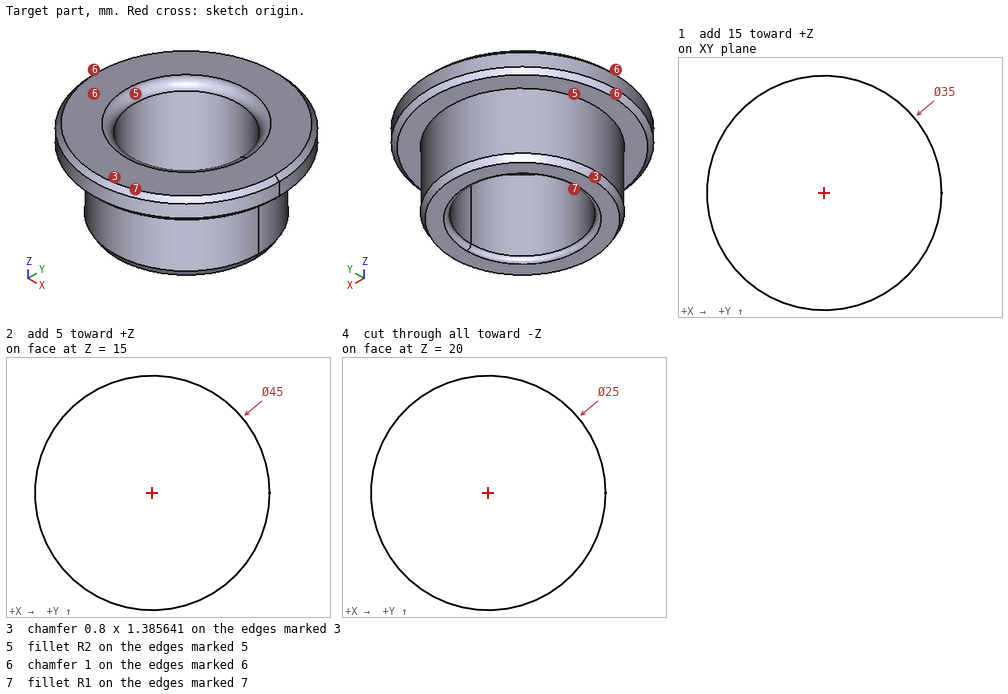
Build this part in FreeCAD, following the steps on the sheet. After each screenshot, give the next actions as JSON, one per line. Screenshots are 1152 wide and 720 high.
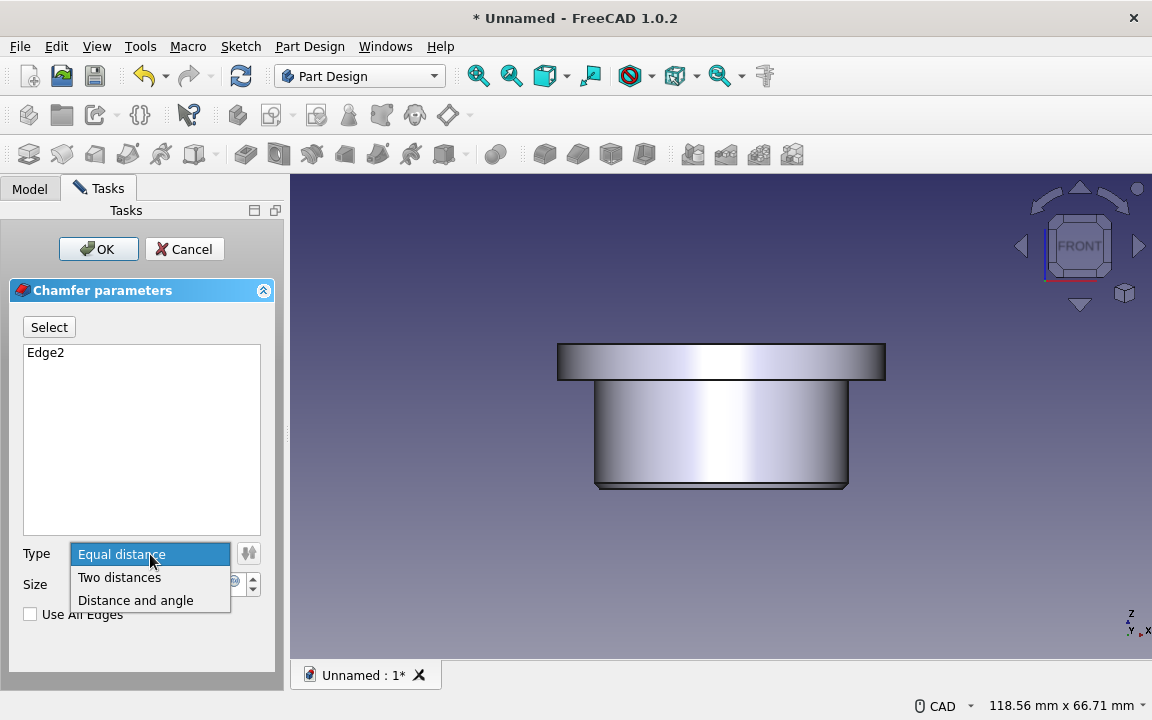
{"action": "left_click", "coordinate": [148, 578]}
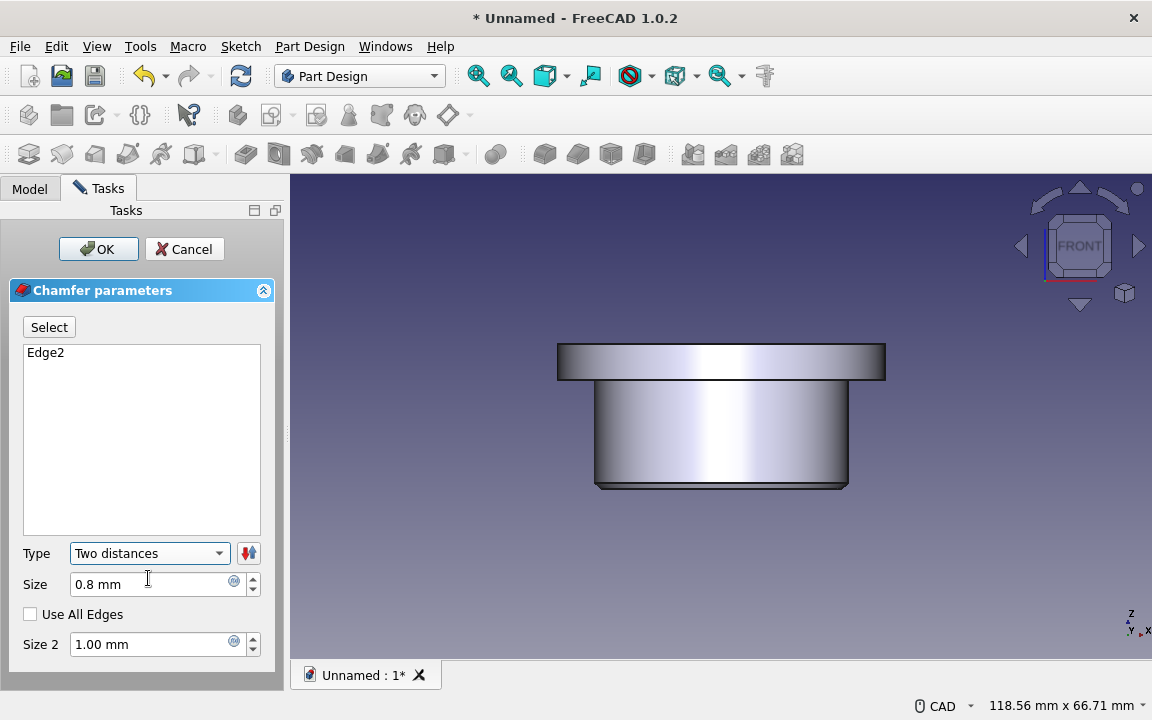
{"action": "triple_click", "coordinate": [158, 644]}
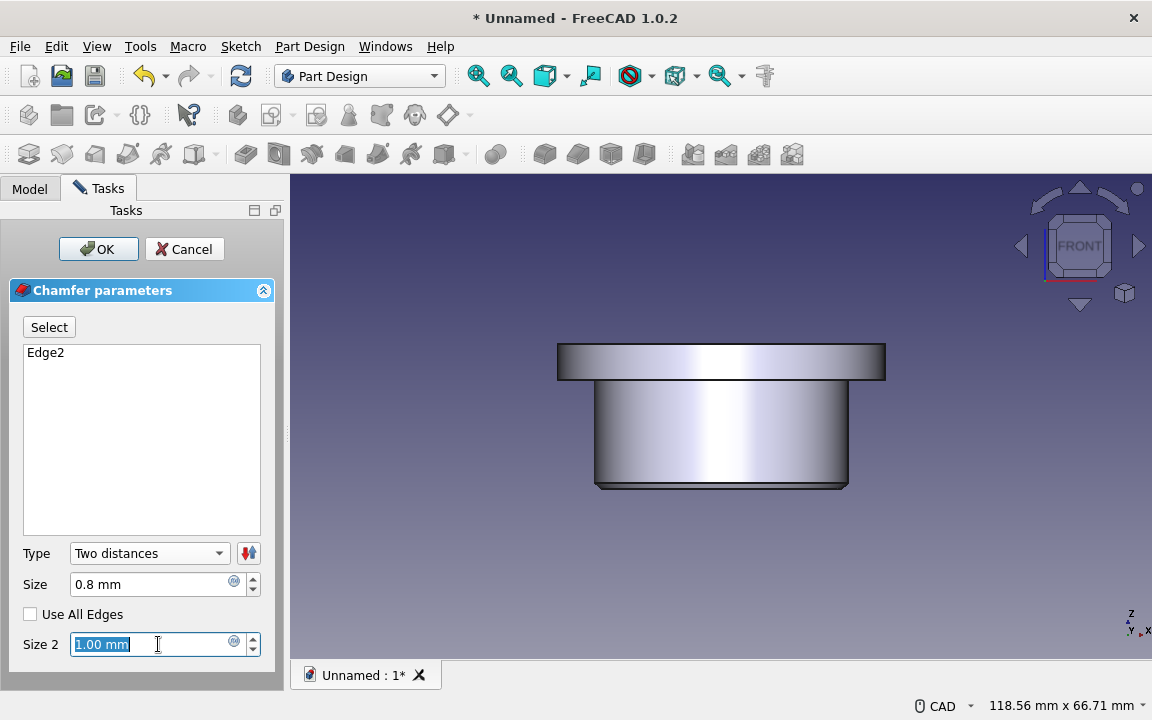
{"action": "type", "text": "1.385641"}
{"action": "key", "text": "Tab"}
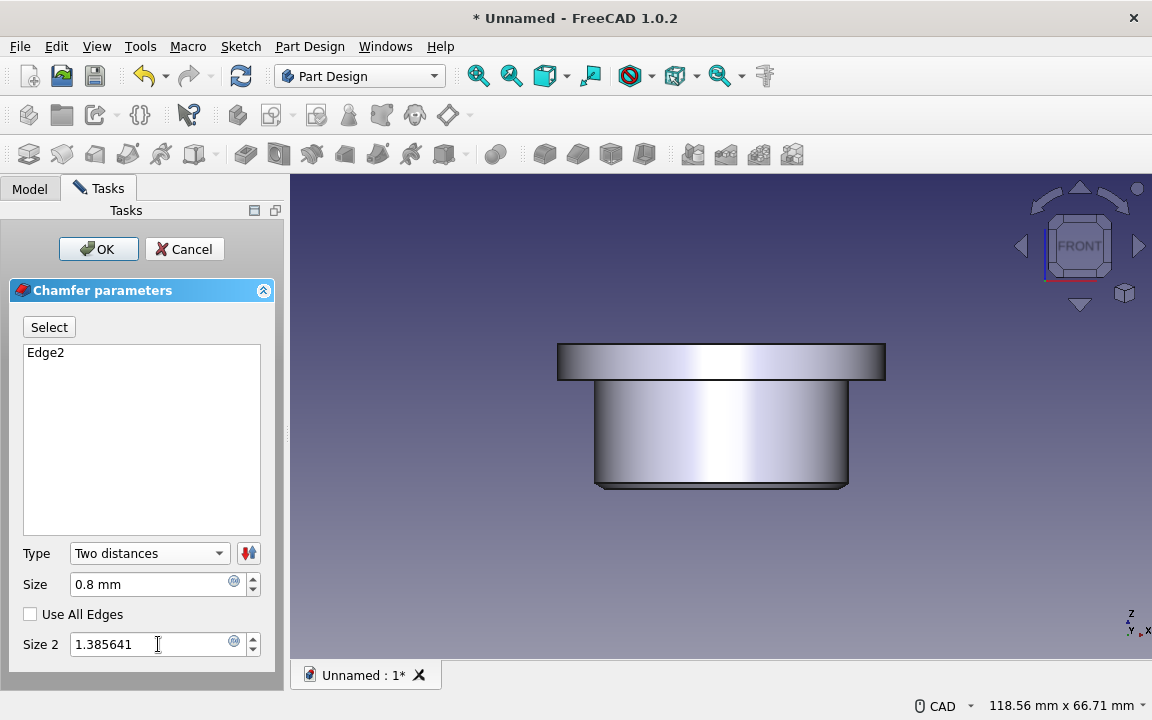
{"action": "left_click", "coordinate": [249, 554]}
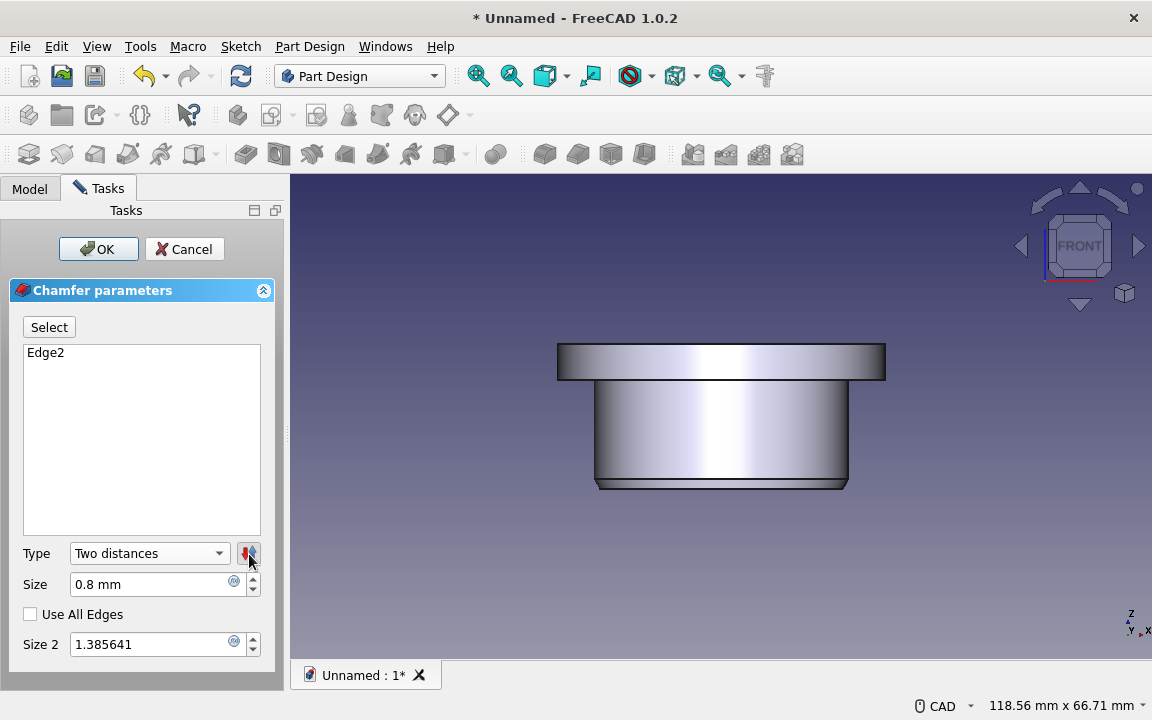
{"action": "left_click", "coordinate": [99, 249]}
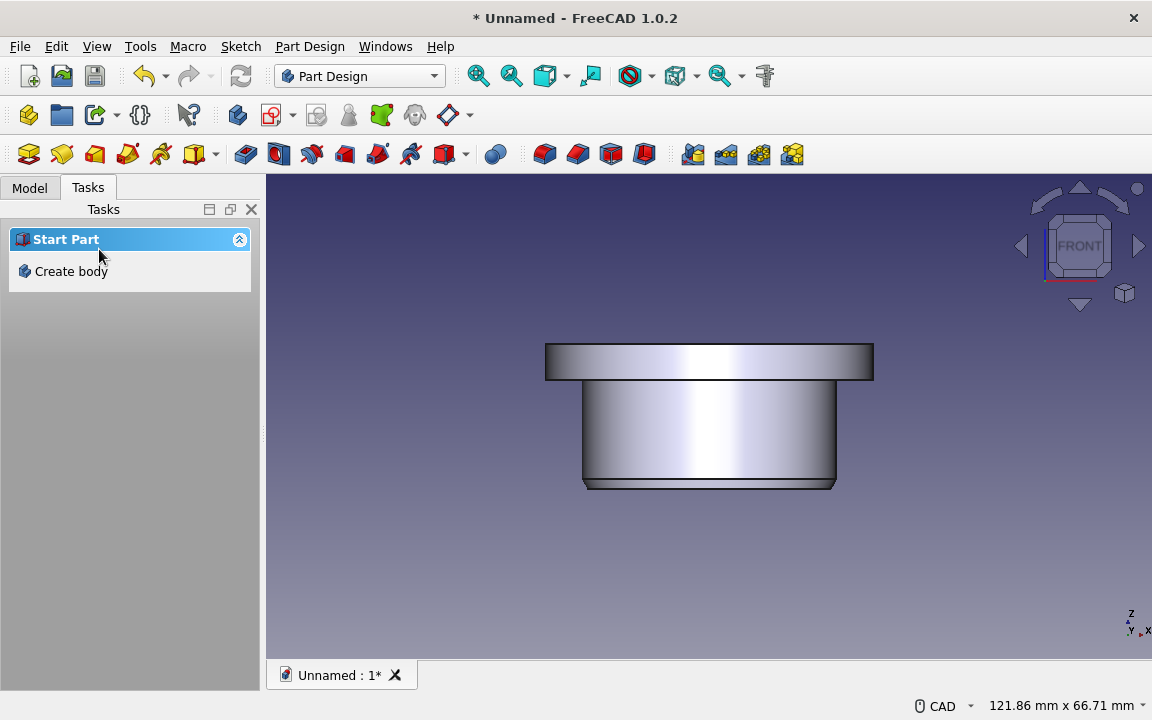
{"action": "key", "text": "v f"}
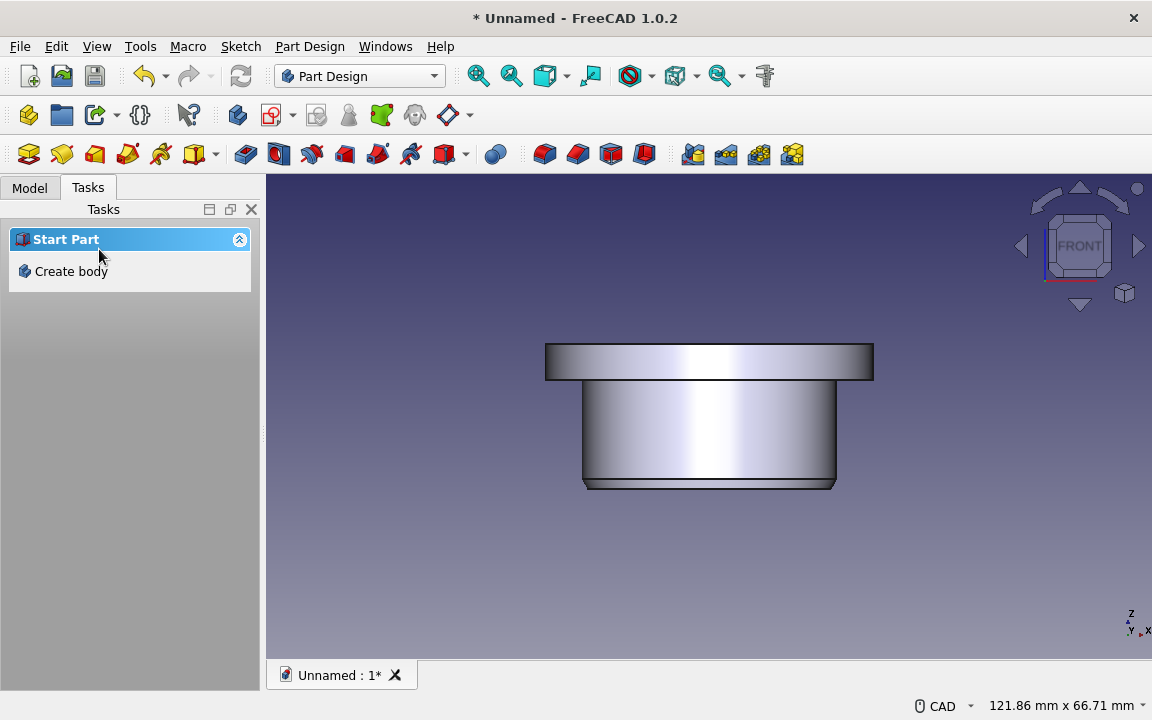
{"action": "key", "text": "0"}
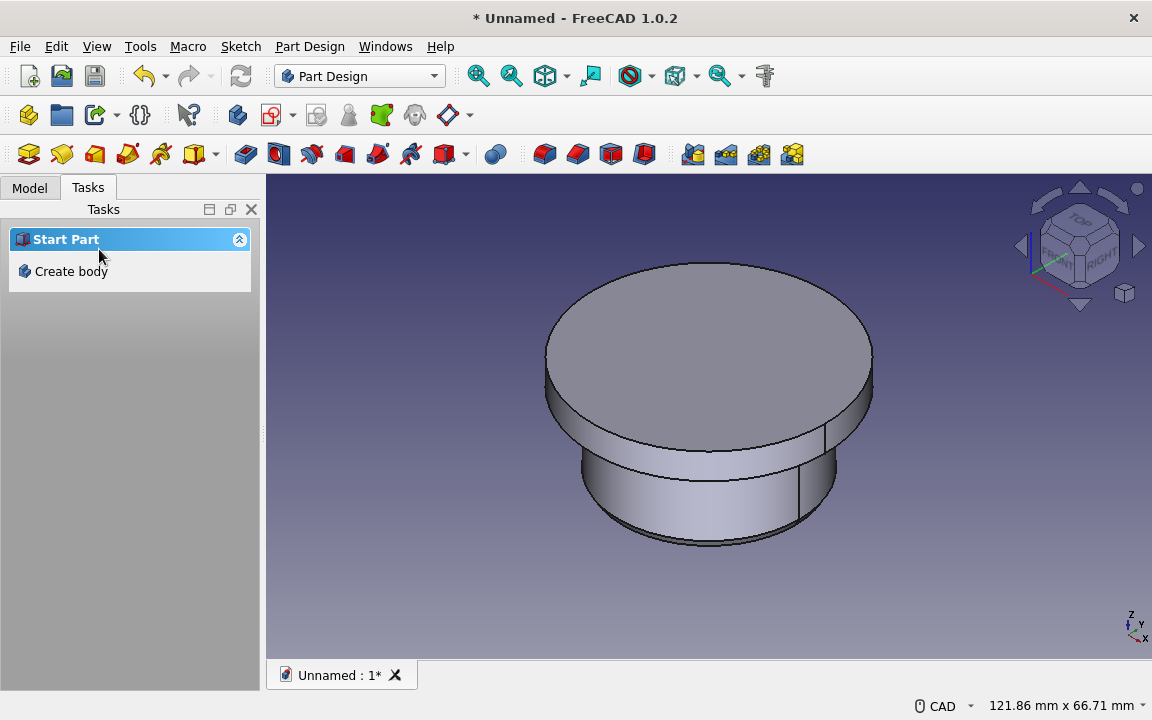
{"action": "left_click", "coordinate": [709, 356]}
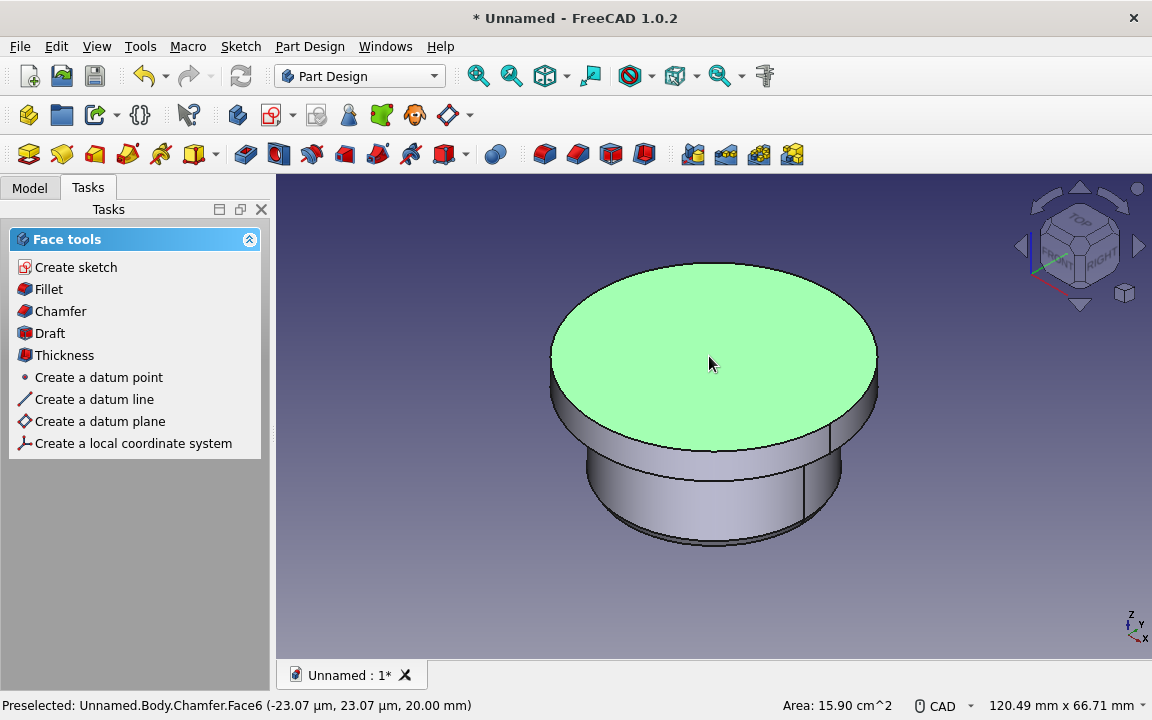
{"action": "left_click", "coordinate": [270, 116]}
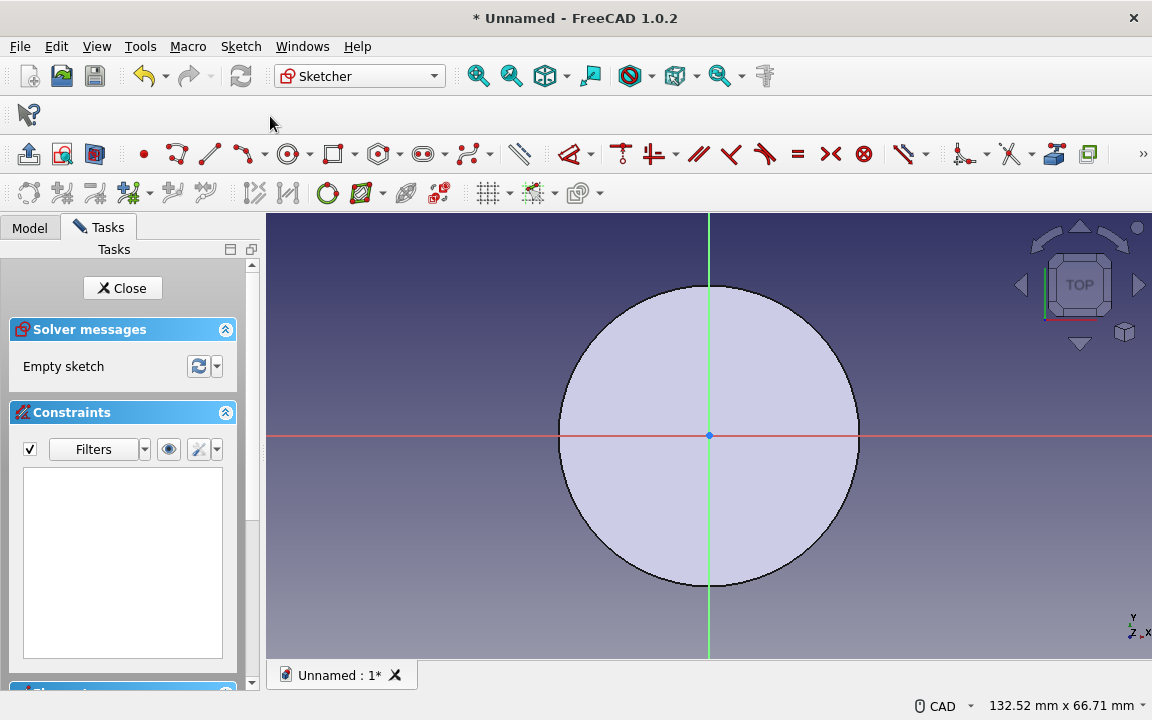
{"action": "scroll", "coordinate": [848, 436], "scroll_direction": "up", "scroll_amount": 2}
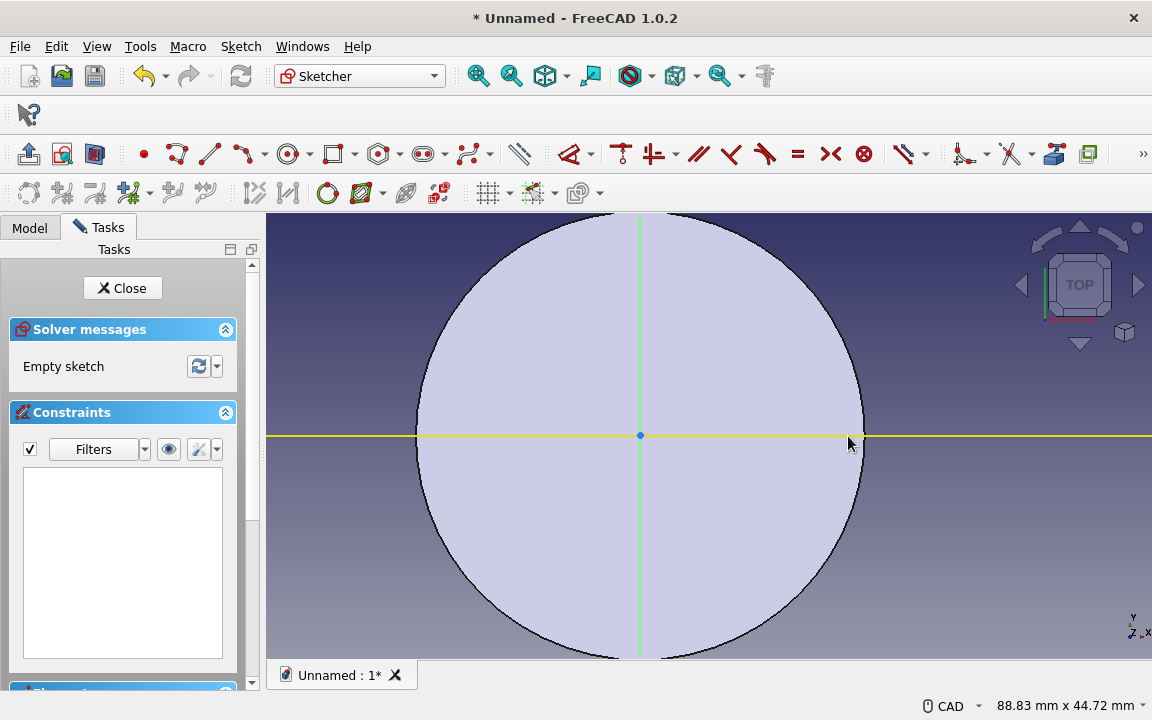
{"action": "left_click", "coordinate": [288, 154]}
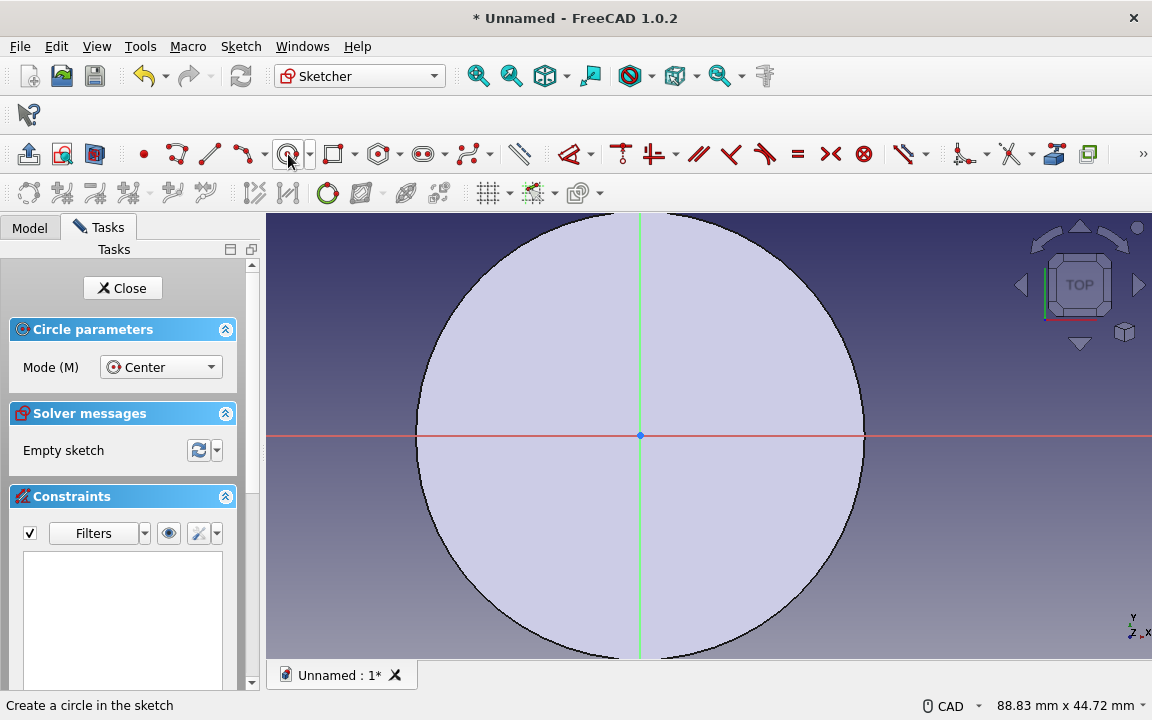
{"action": "left_click", "coordinate": [640, 436]}
{"action": "left_click", "coordinate": [728, 348]}
{"action": "key", "text": "Escape"}